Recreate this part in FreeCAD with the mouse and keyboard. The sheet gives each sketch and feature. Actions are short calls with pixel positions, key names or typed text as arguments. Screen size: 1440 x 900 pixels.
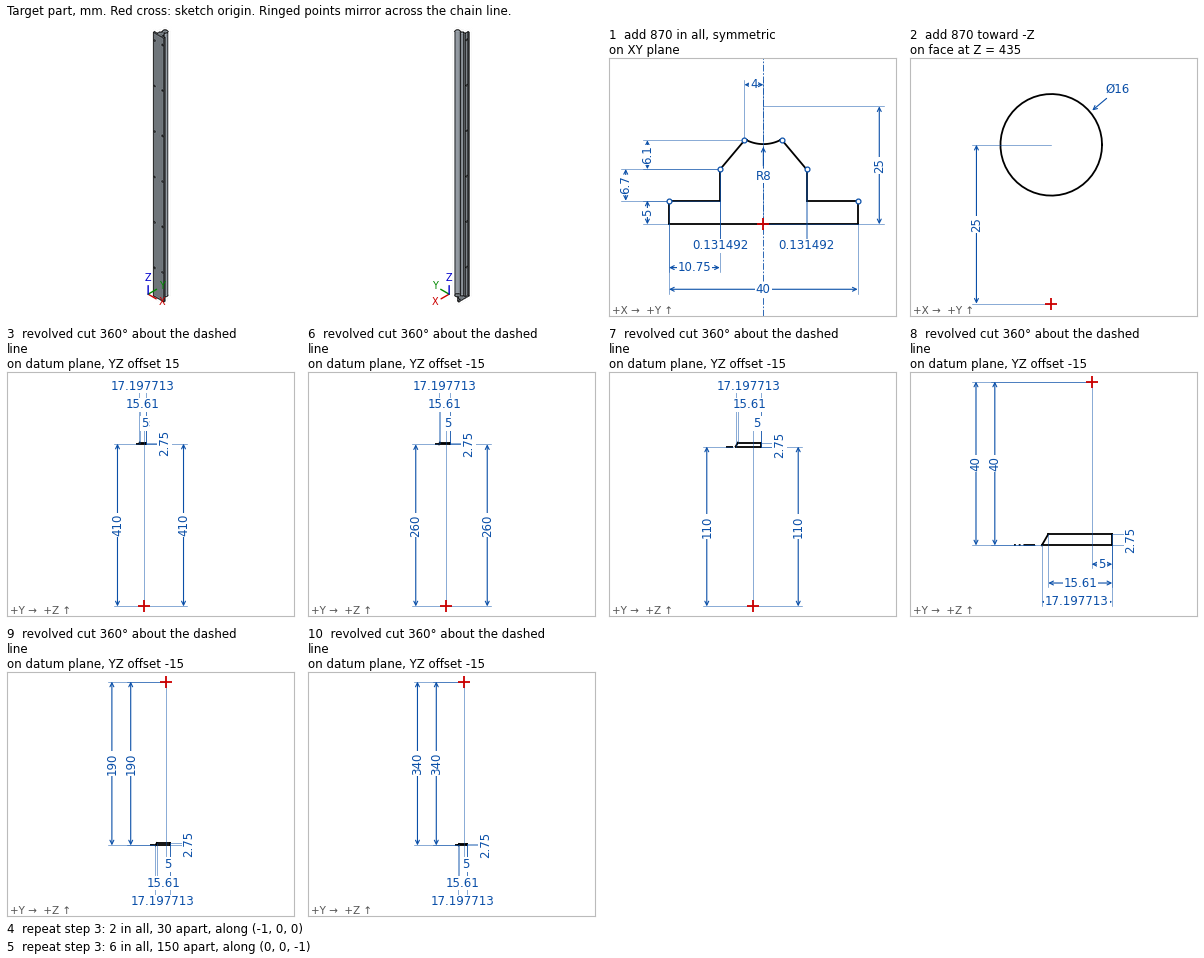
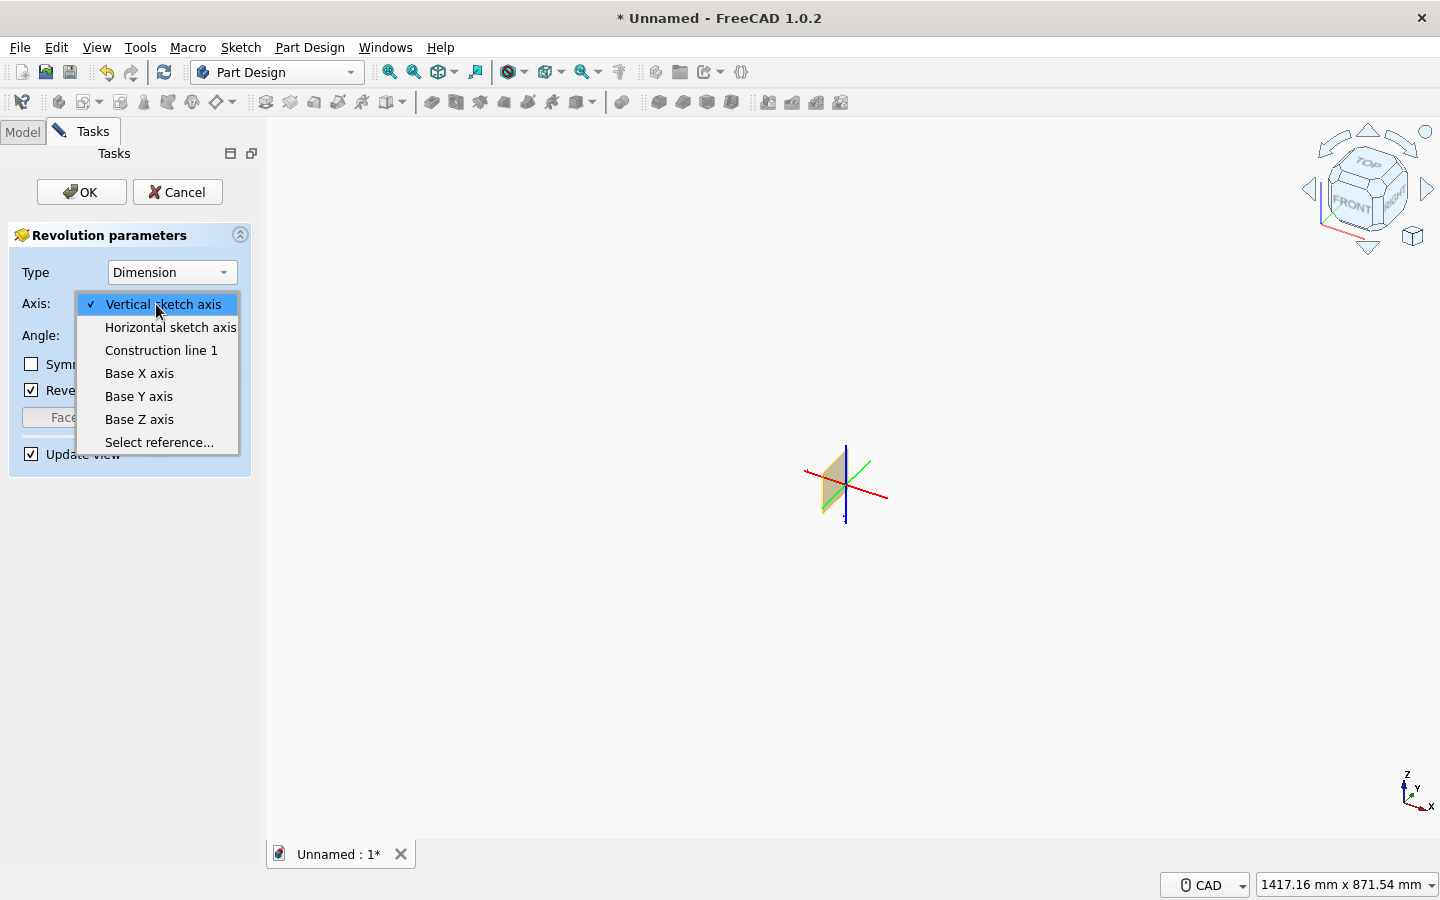
click(156, 350)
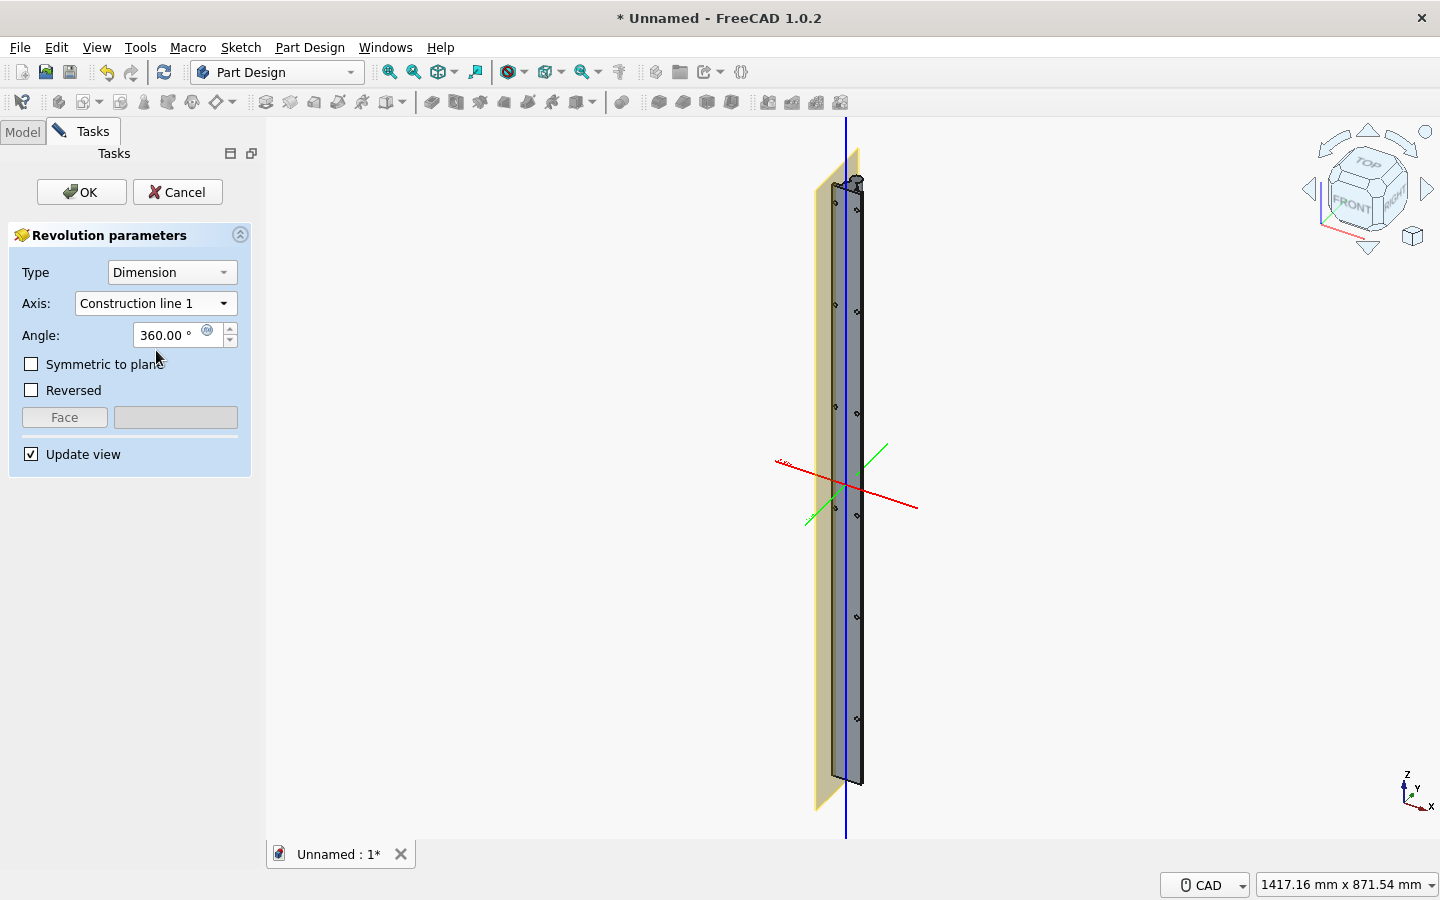
click(82, 192)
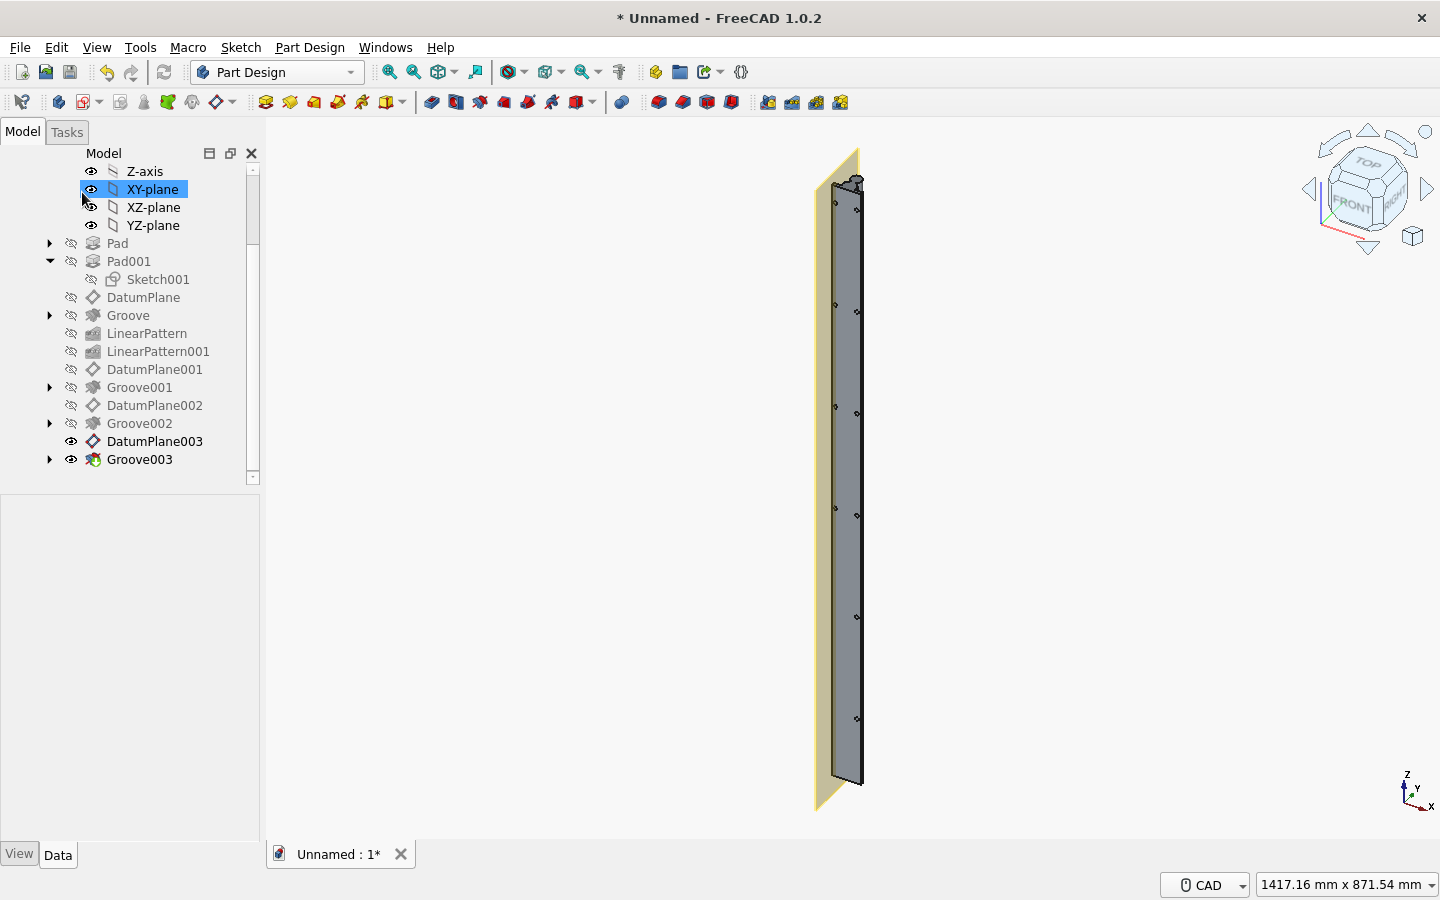
click(116, 441)
key(space)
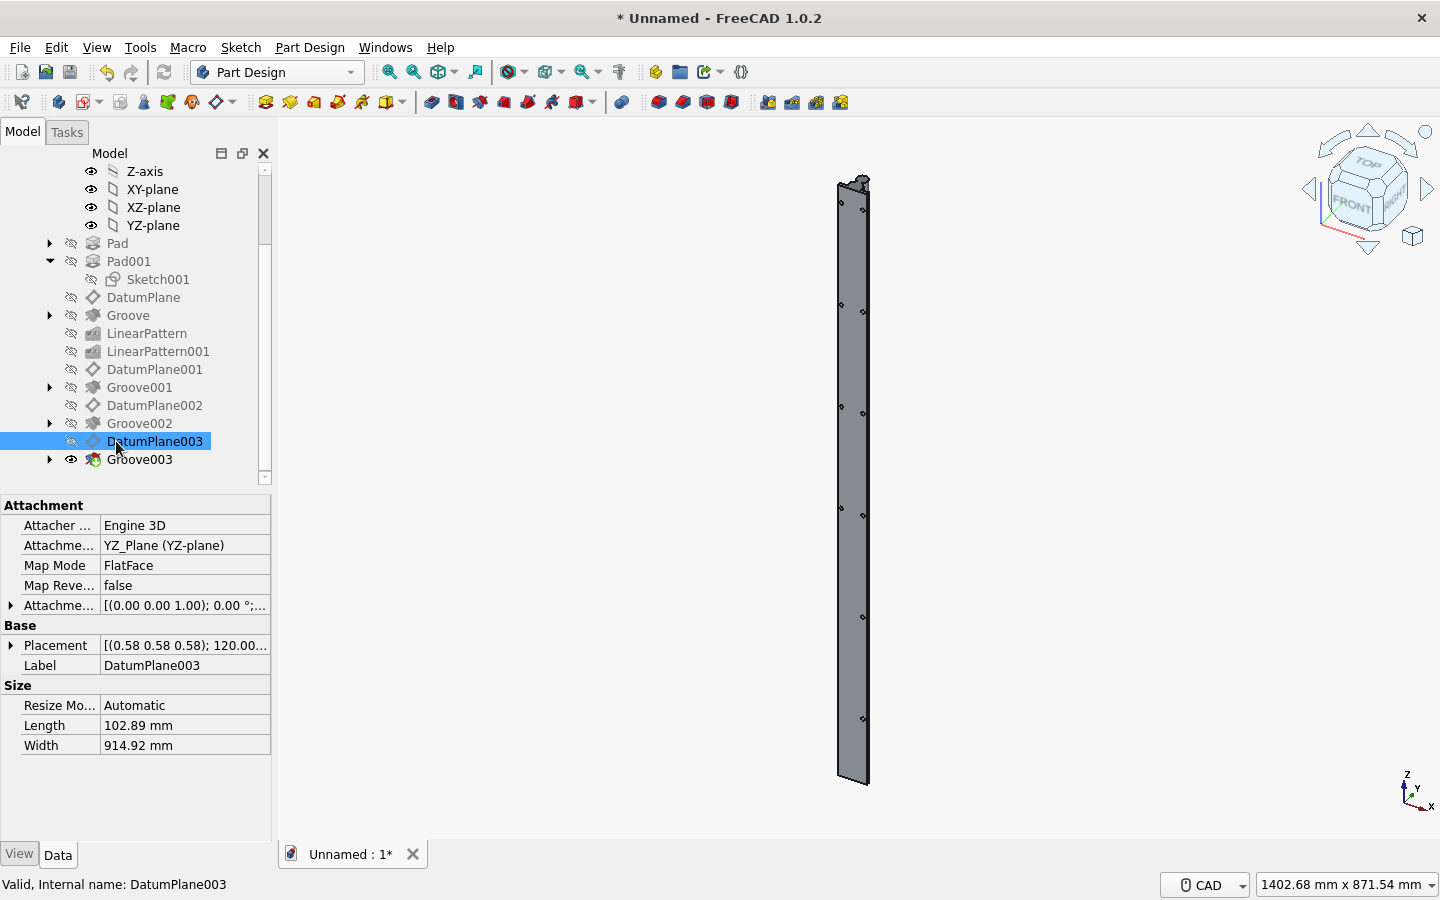
scroll(160, 311, down, 3)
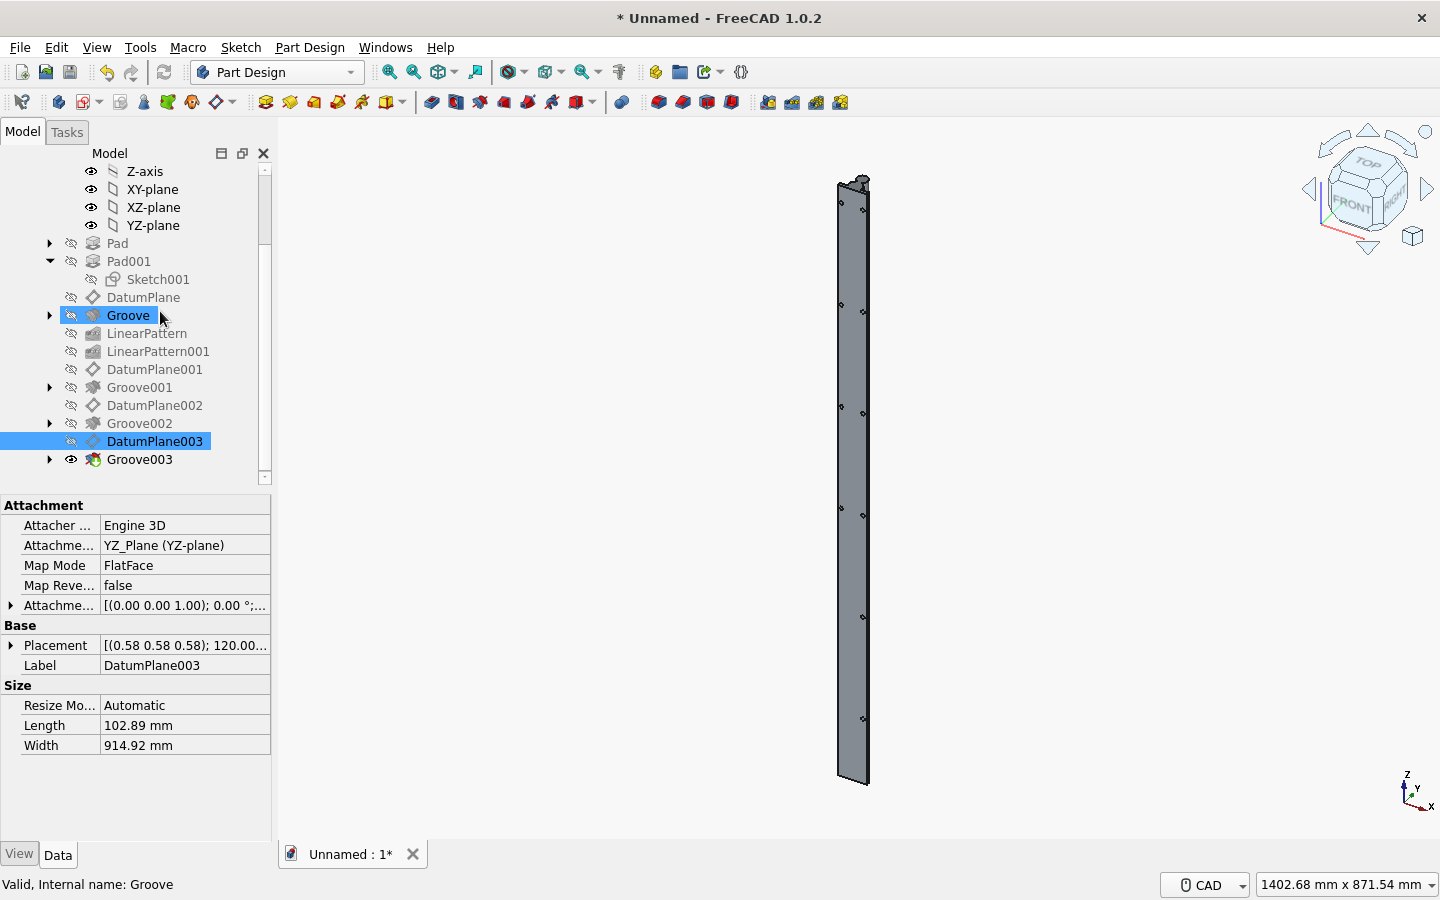
scroll(160, 311, up, 15)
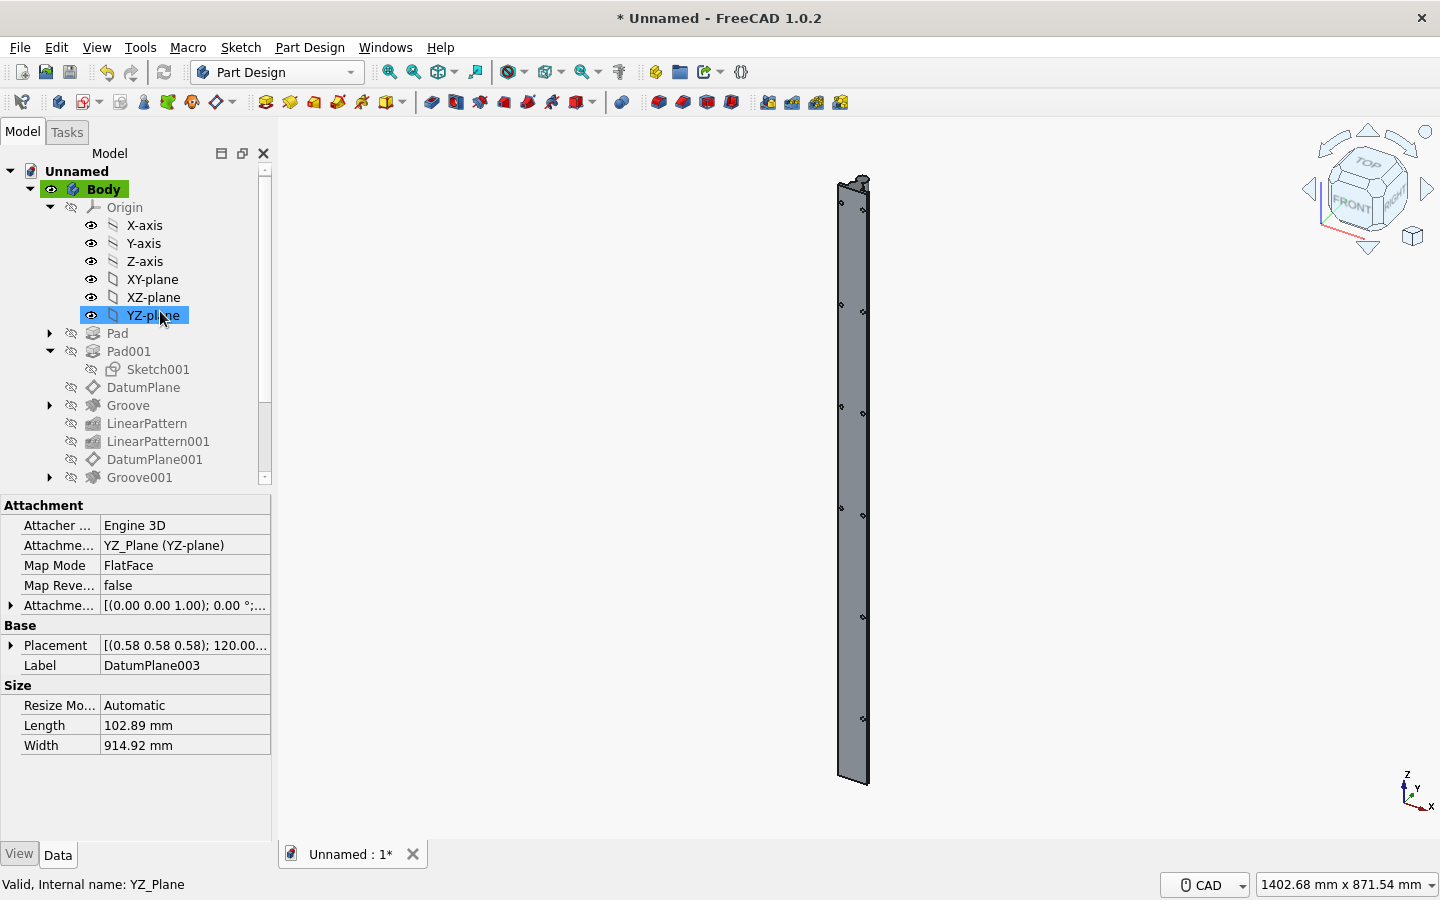
click(136, 315)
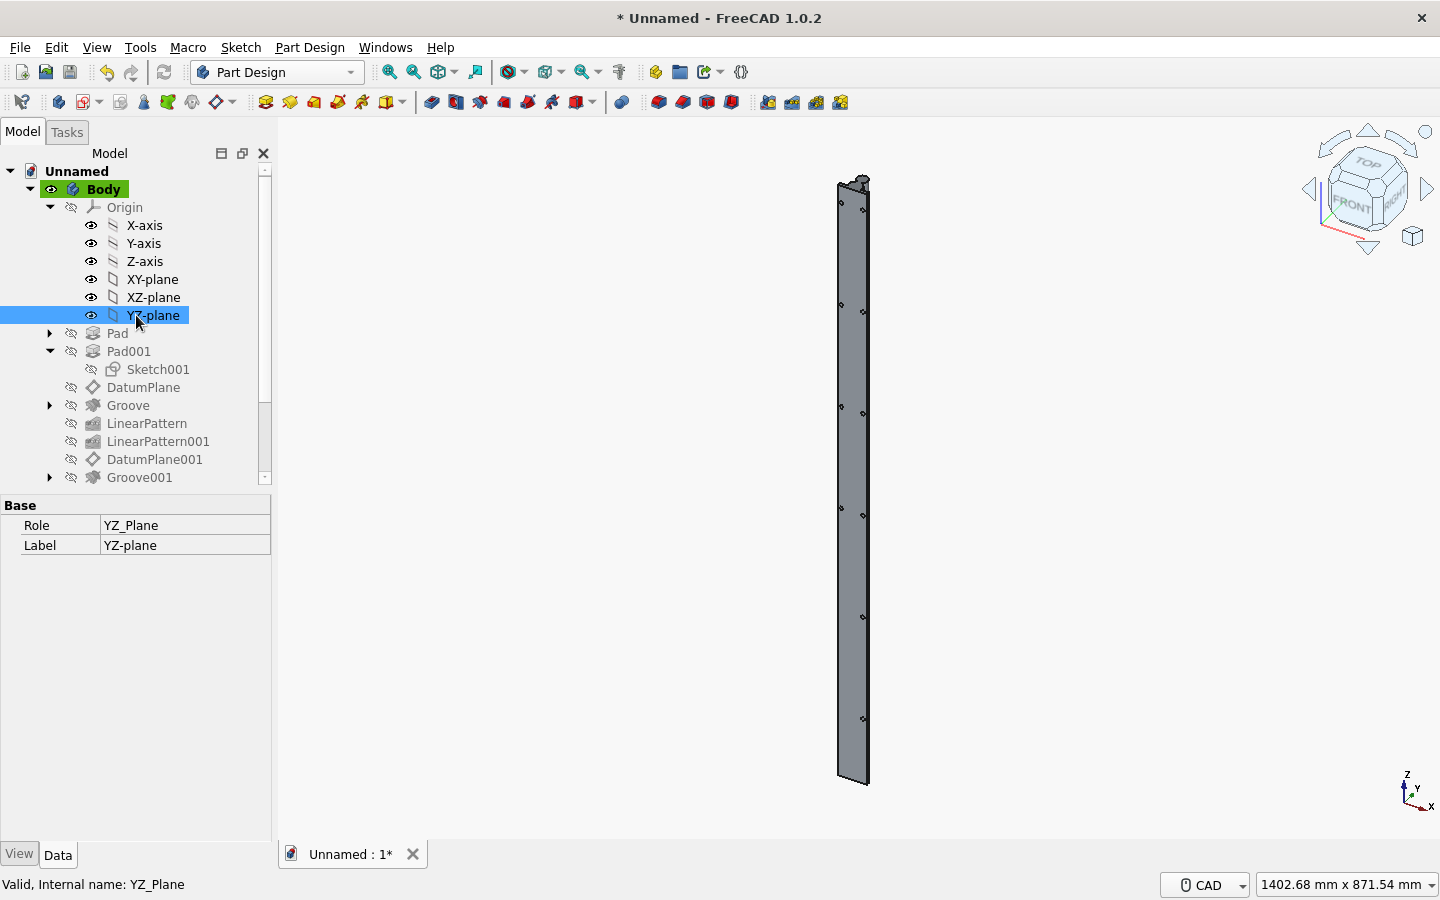
click(216, 102)